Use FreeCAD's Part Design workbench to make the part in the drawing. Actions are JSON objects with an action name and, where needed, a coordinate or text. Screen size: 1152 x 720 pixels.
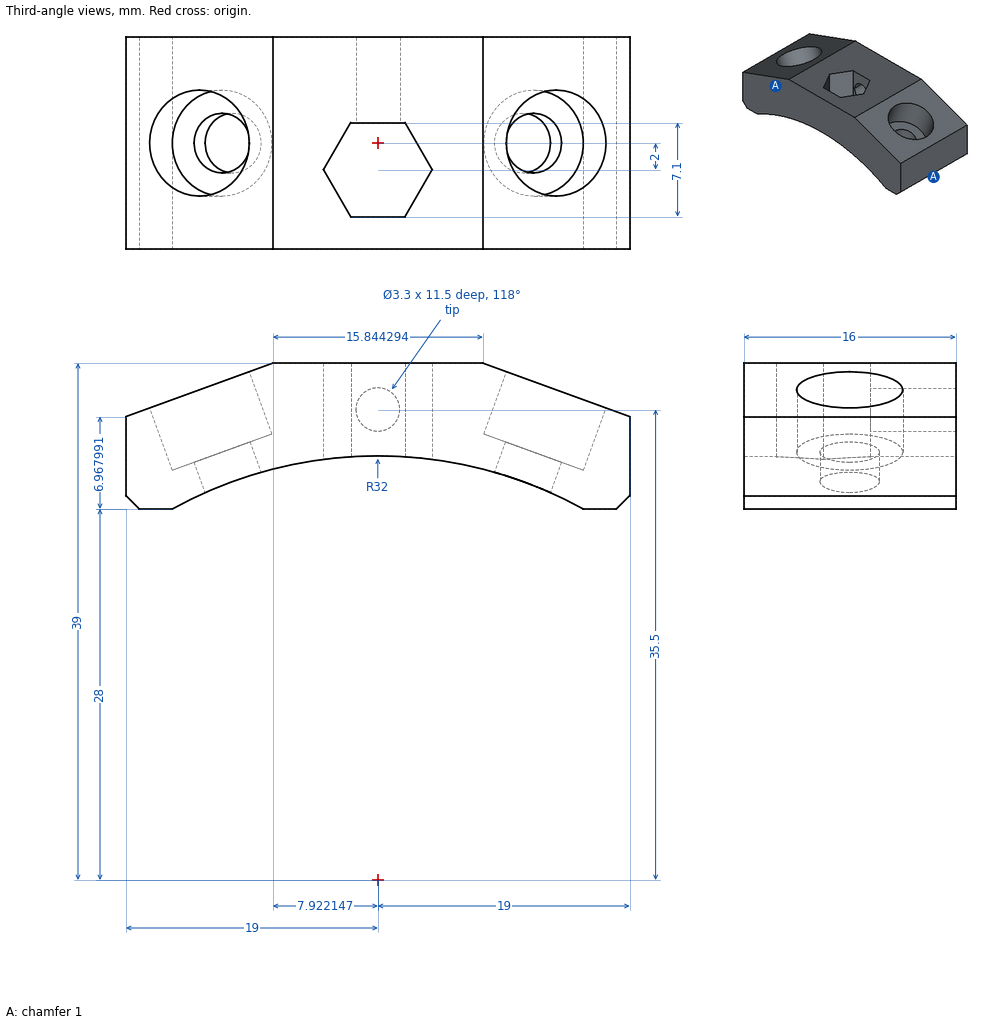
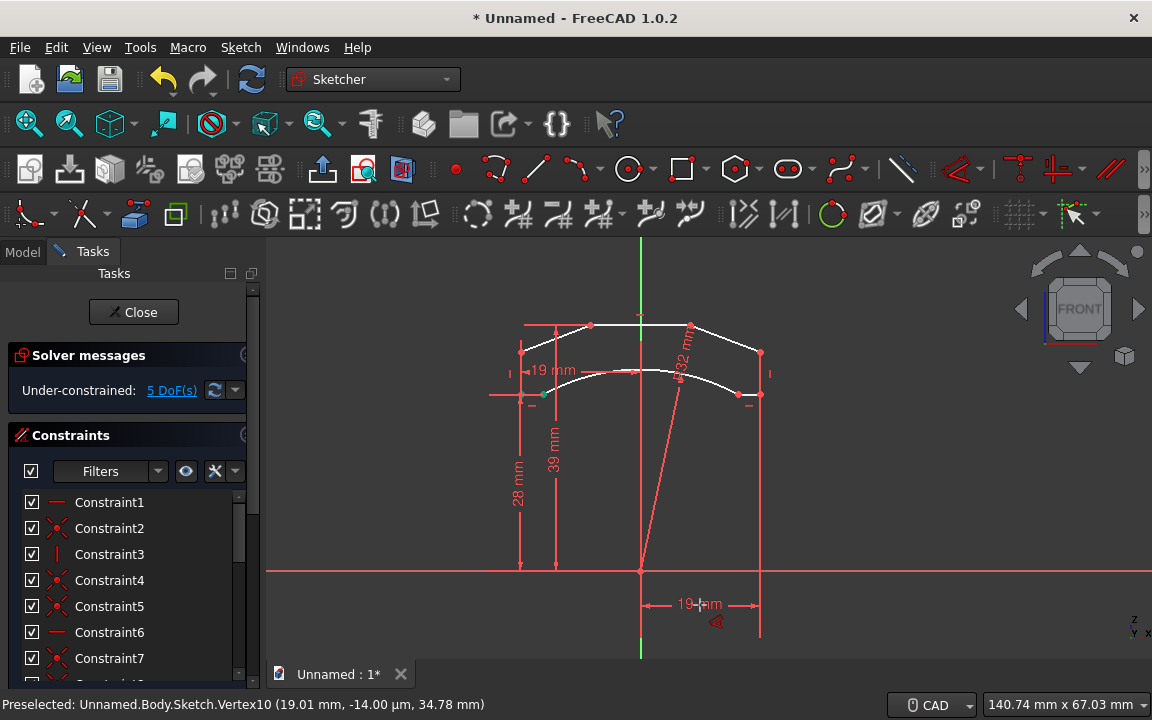
{"action": "left_click", "coordinate": [760, 395]}
{"action": "left_click", "coordinate": [794, 483]}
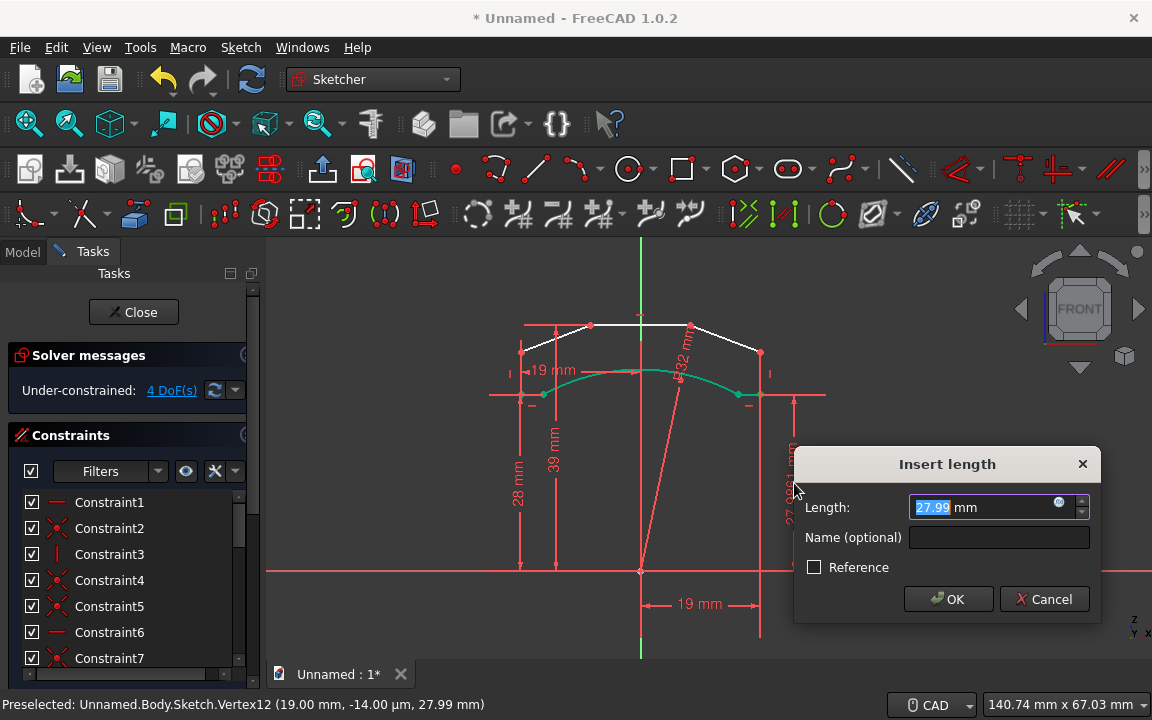
{"action": "type", "text": "28"}
{"action": "key", "text": "Return"}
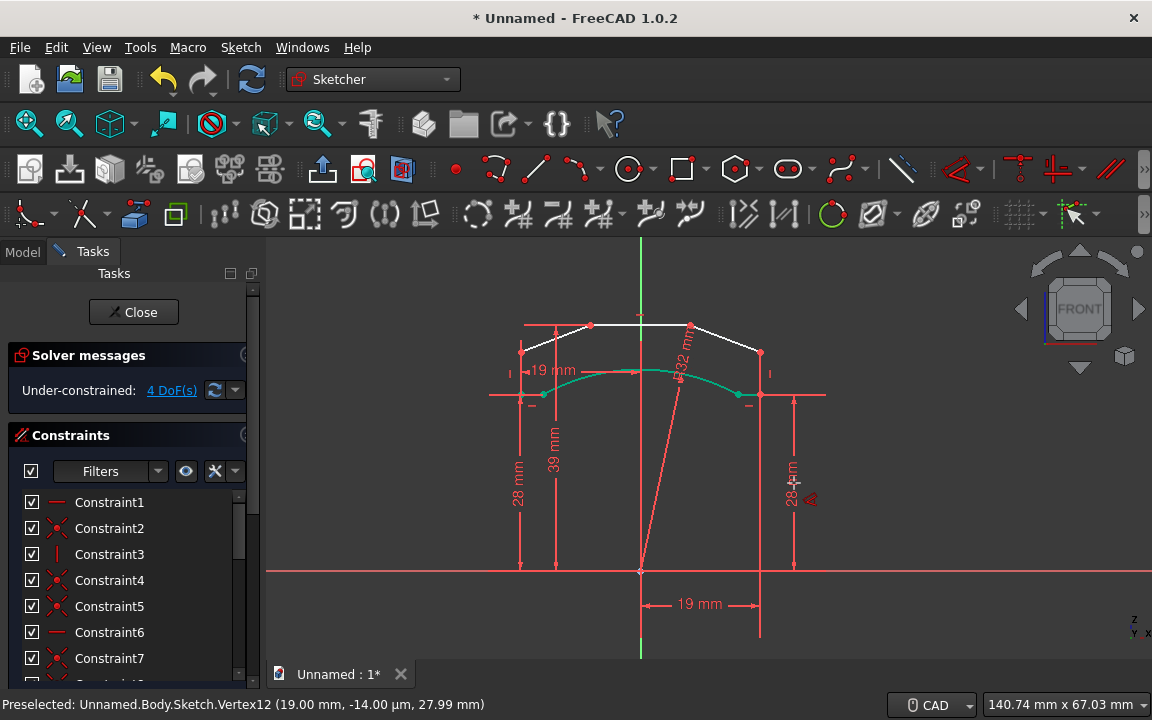
{"action": "left_click", "coordinate": [521, 382]}
{"action": "left_click", "coordinate": [463, 373]}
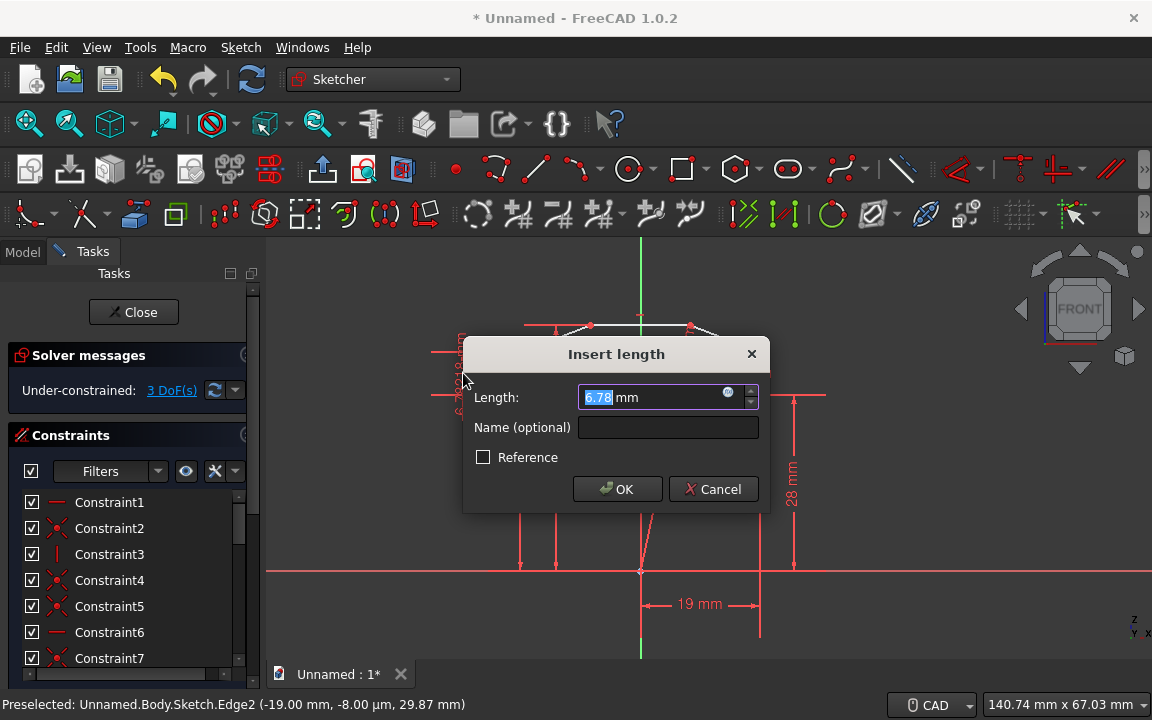
{"action": "type", "text": "6.967991"}
{"action": "key", "text": "Return"}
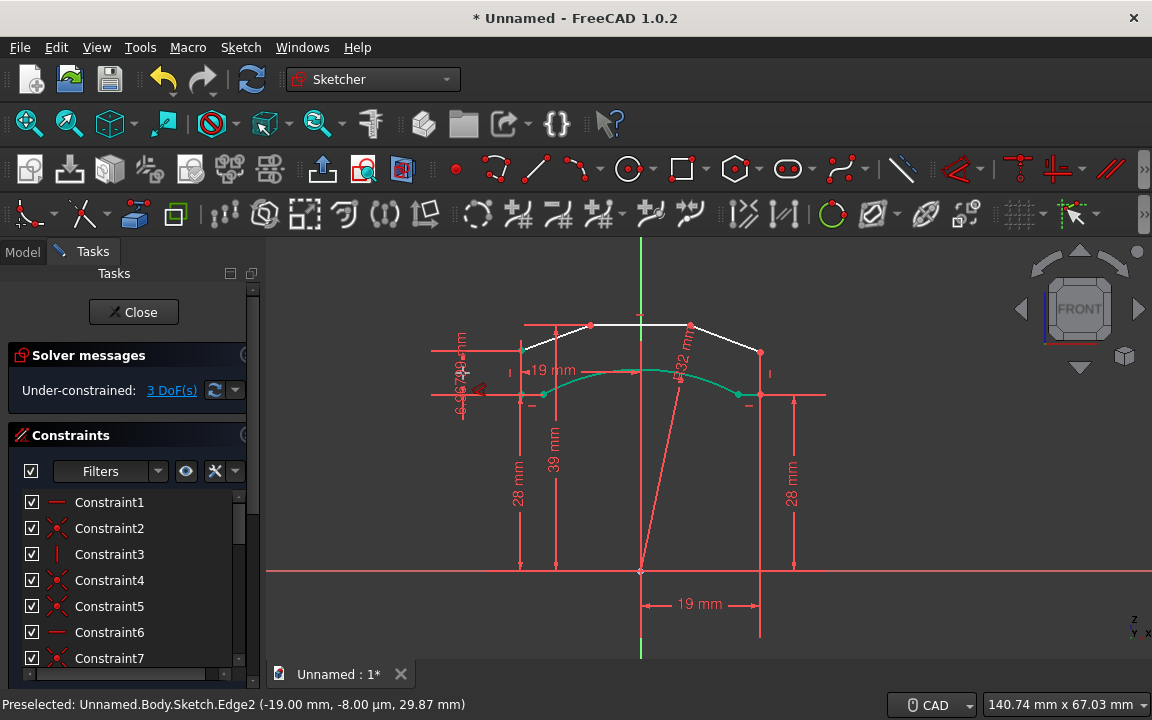
{"action": "left_click", "coordinate": [760, 365]}
{"action": "left_click", "coordinate": [794, 373]}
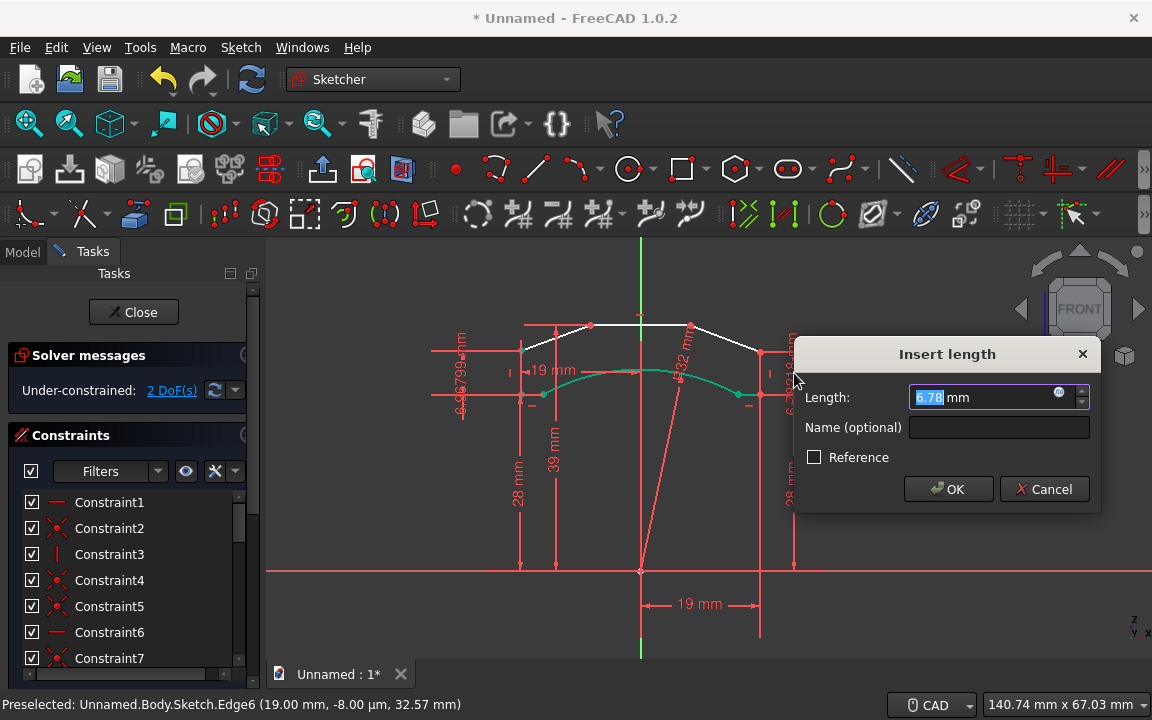
{"action": "type", "text": "6.967991"}
{"action": "key", "text": "Return"}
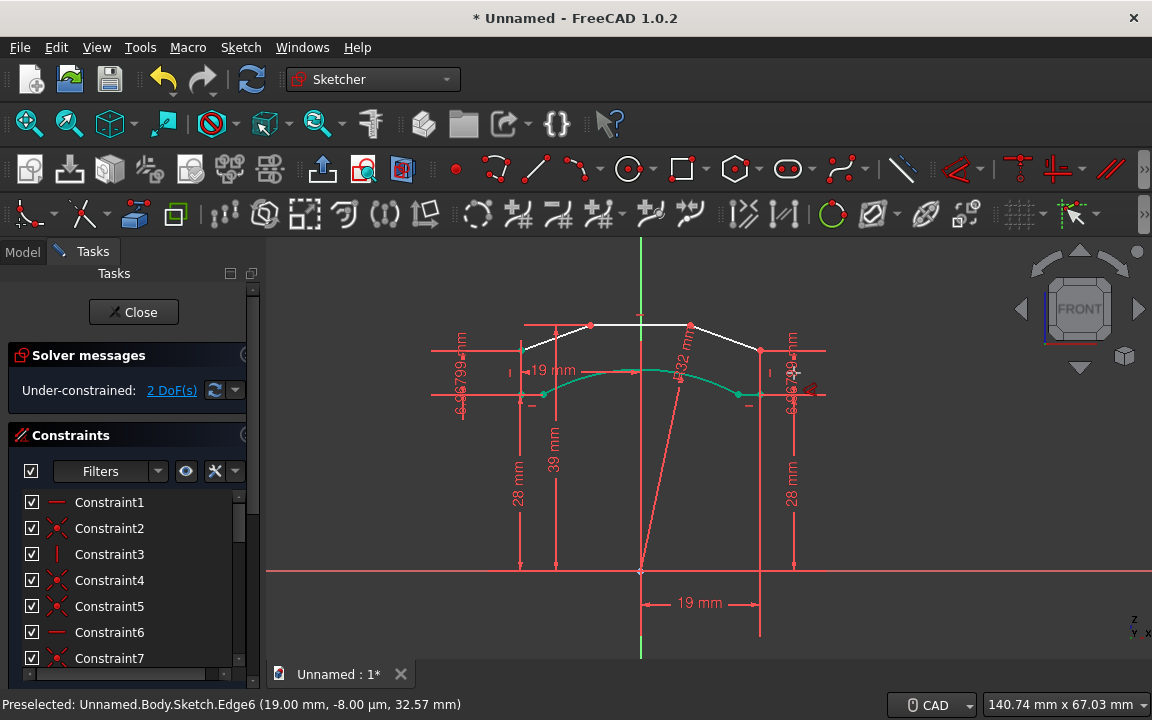
{"action": "left_click", "coordinate": [620, 325]}
{"action": "left_click", "coordinate": [617, 291]}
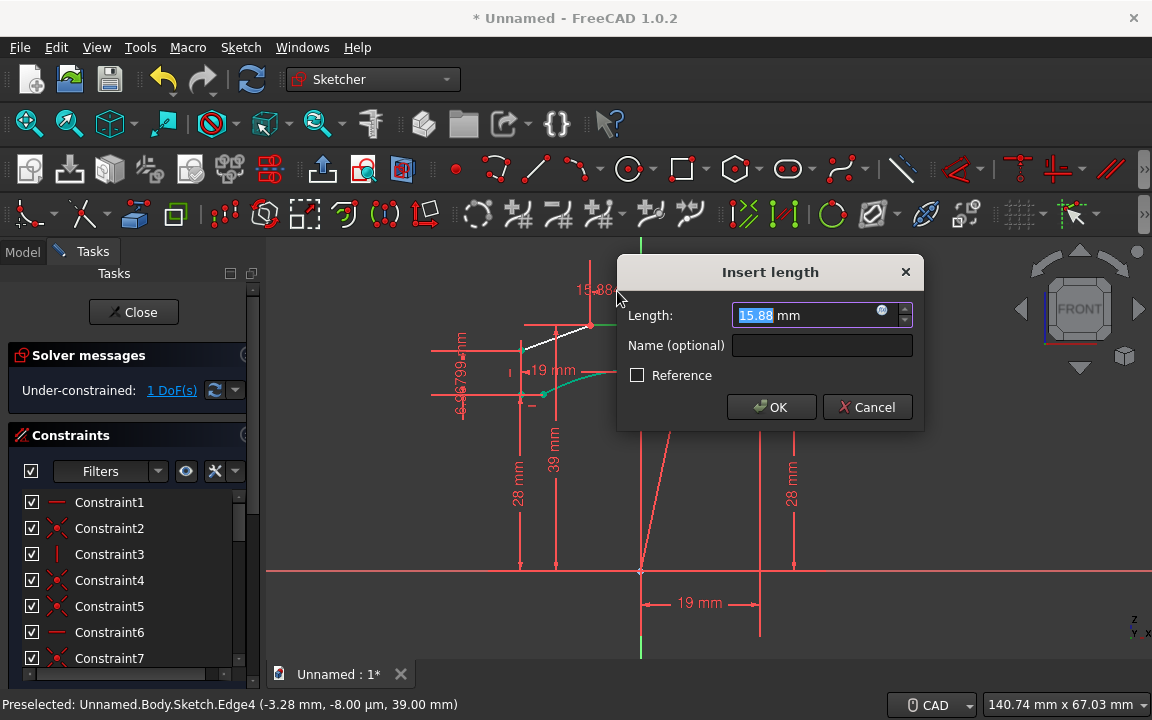
{"action": "type", "text": "15.844294"}
{"action": "key", "text": "Return"}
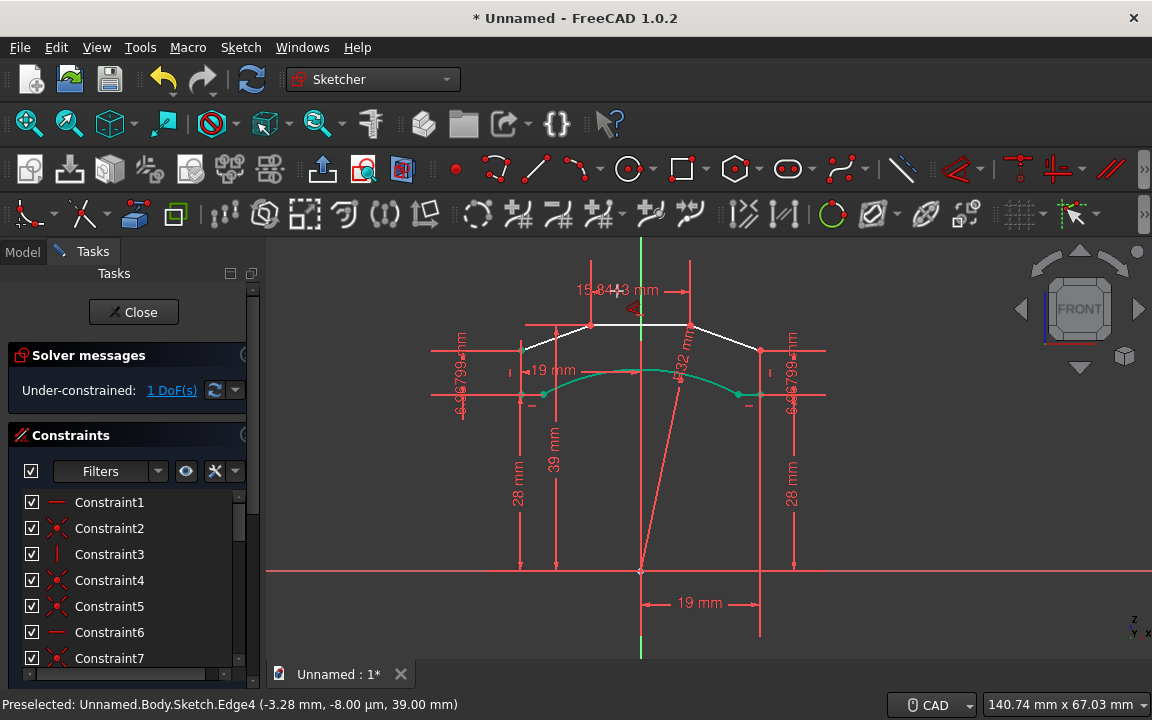
{"action": "left_click", "coordinate": [591, 325]}
{"action": "left_click", "coordinate": [616, 605]}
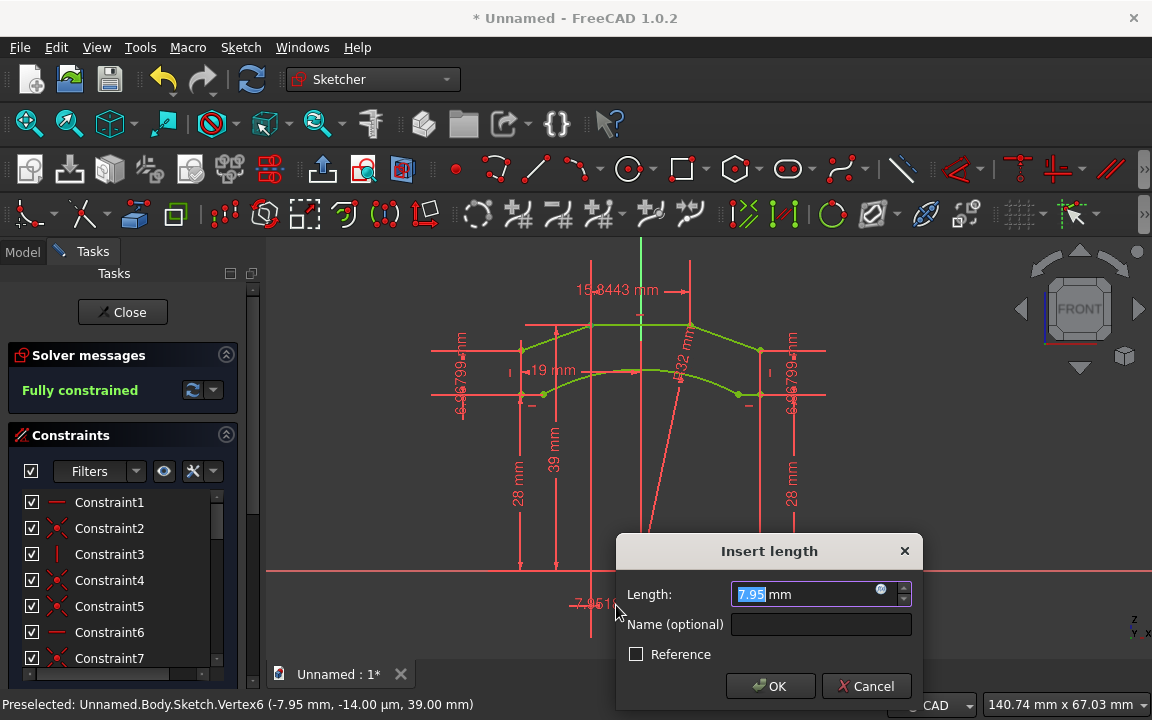
{"action": "type", "text": "7.922147"}
{"action": "key", "text": "Return"}
{"action": "key", "text": "Escape"}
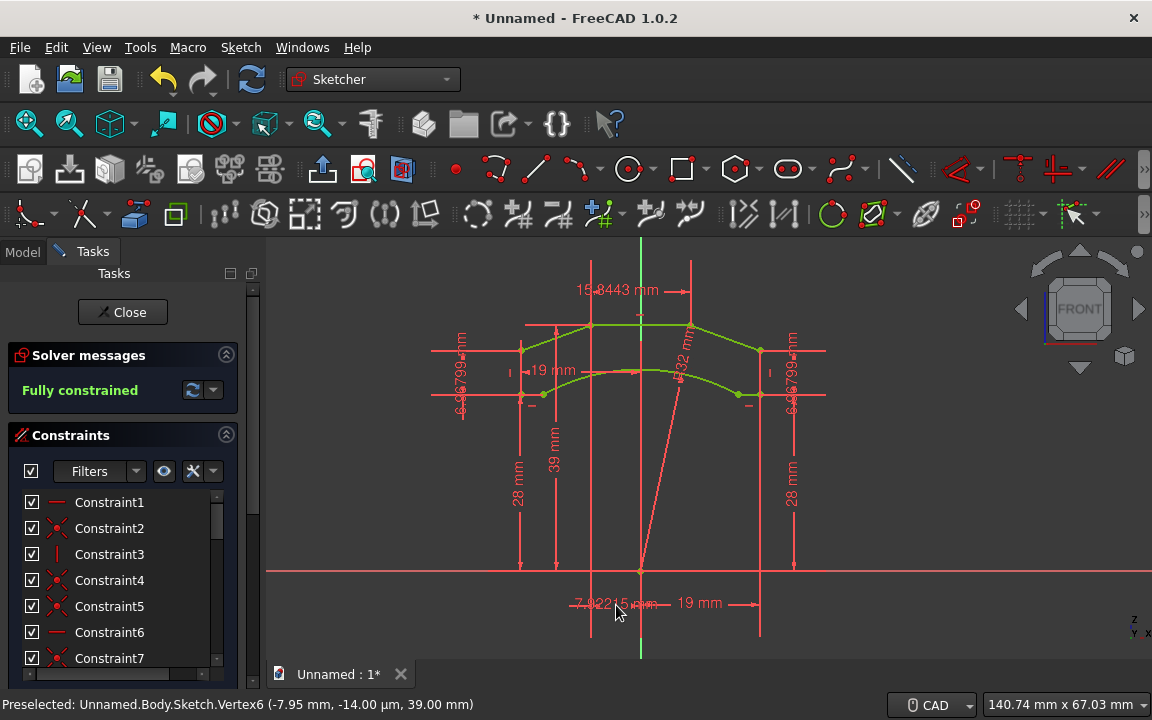
{"action": "left_click", "coordinate": [123, 312]}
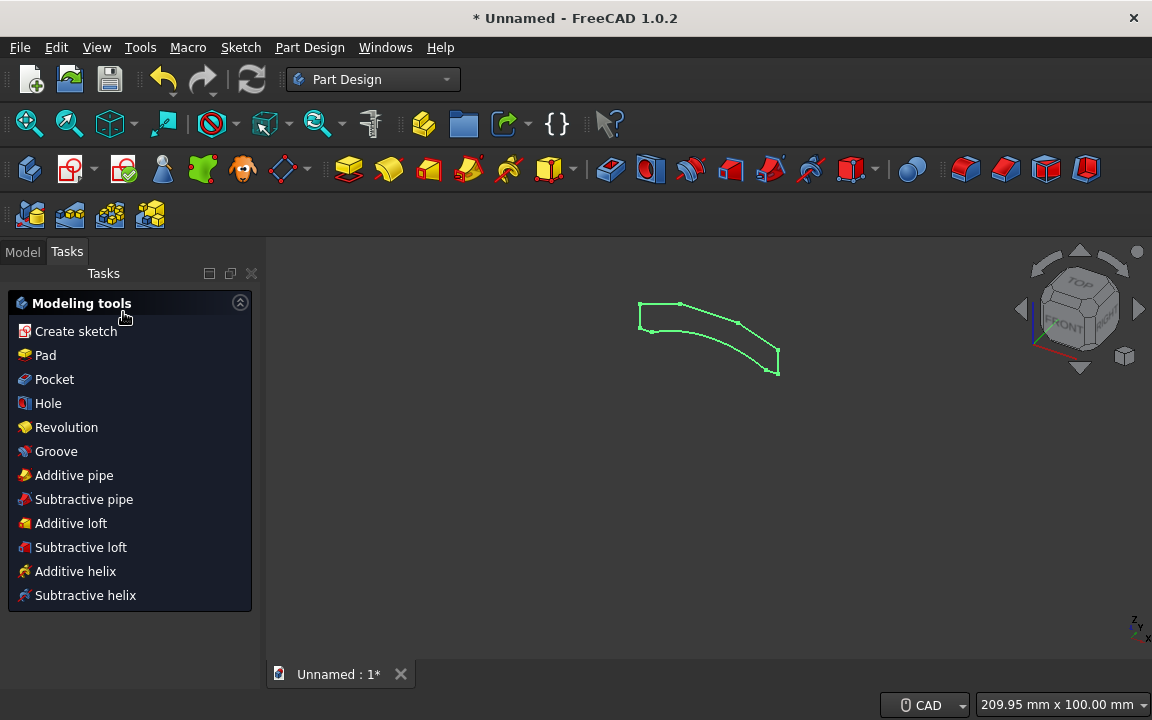
{"action": "left_click", "coordinate": [350, 170]}